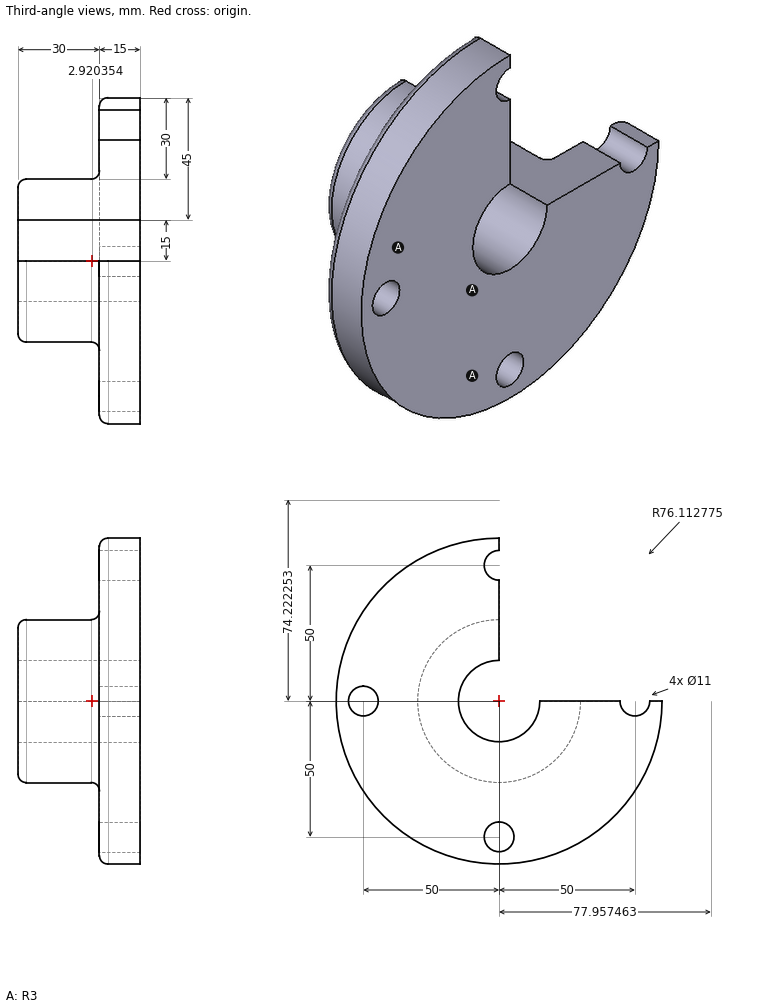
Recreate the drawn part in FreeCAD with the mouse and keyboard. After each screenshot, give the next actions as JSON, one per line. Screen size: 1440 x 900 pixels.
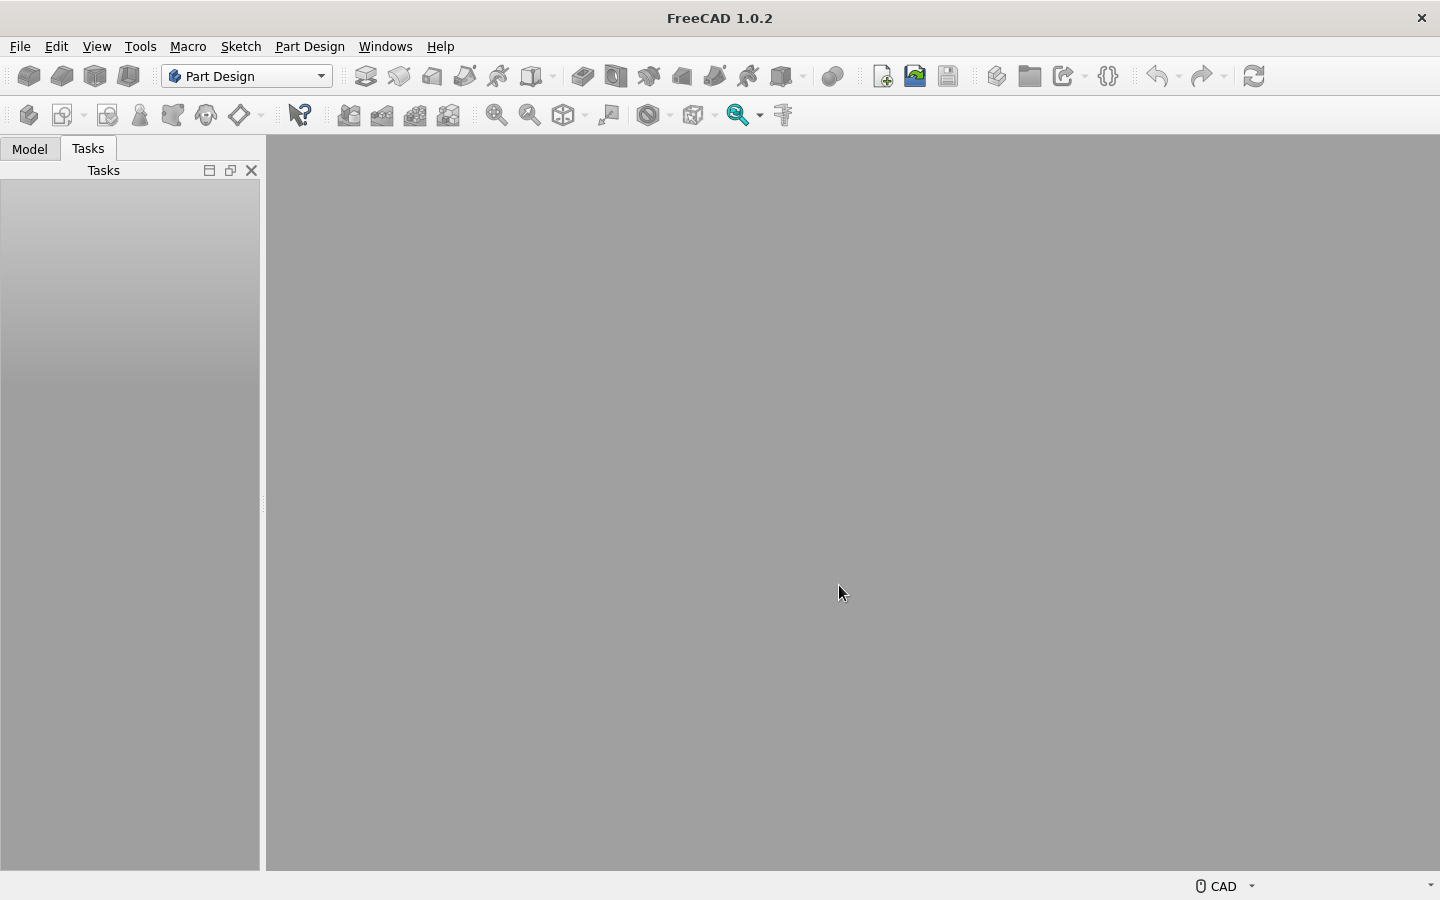
{"action": "left_click", "coordinate": [882, 76]}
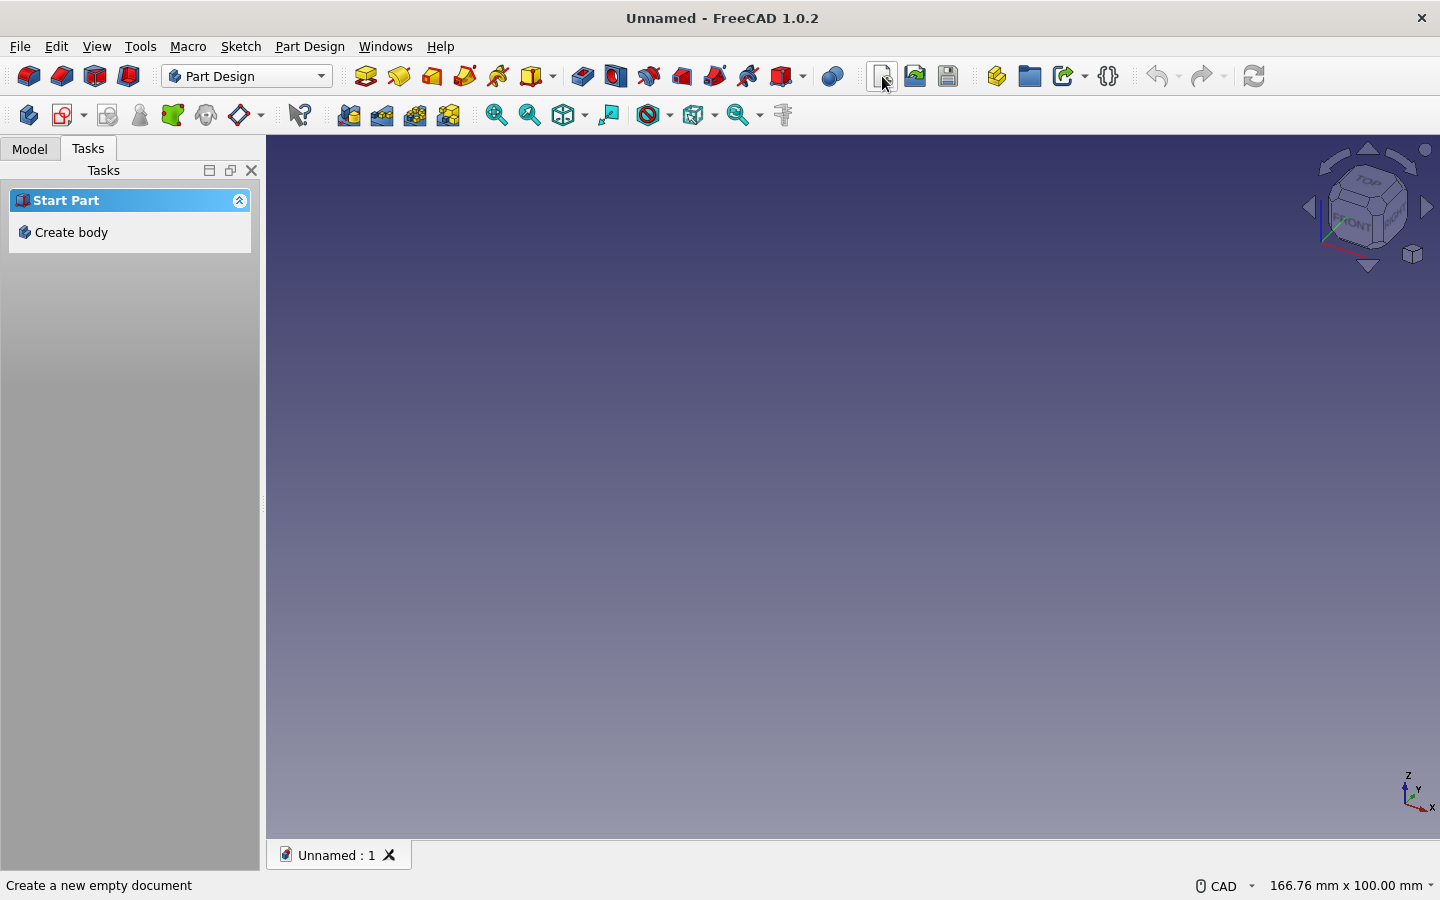
{"action": "left_click", "coordinate": [62, 116]}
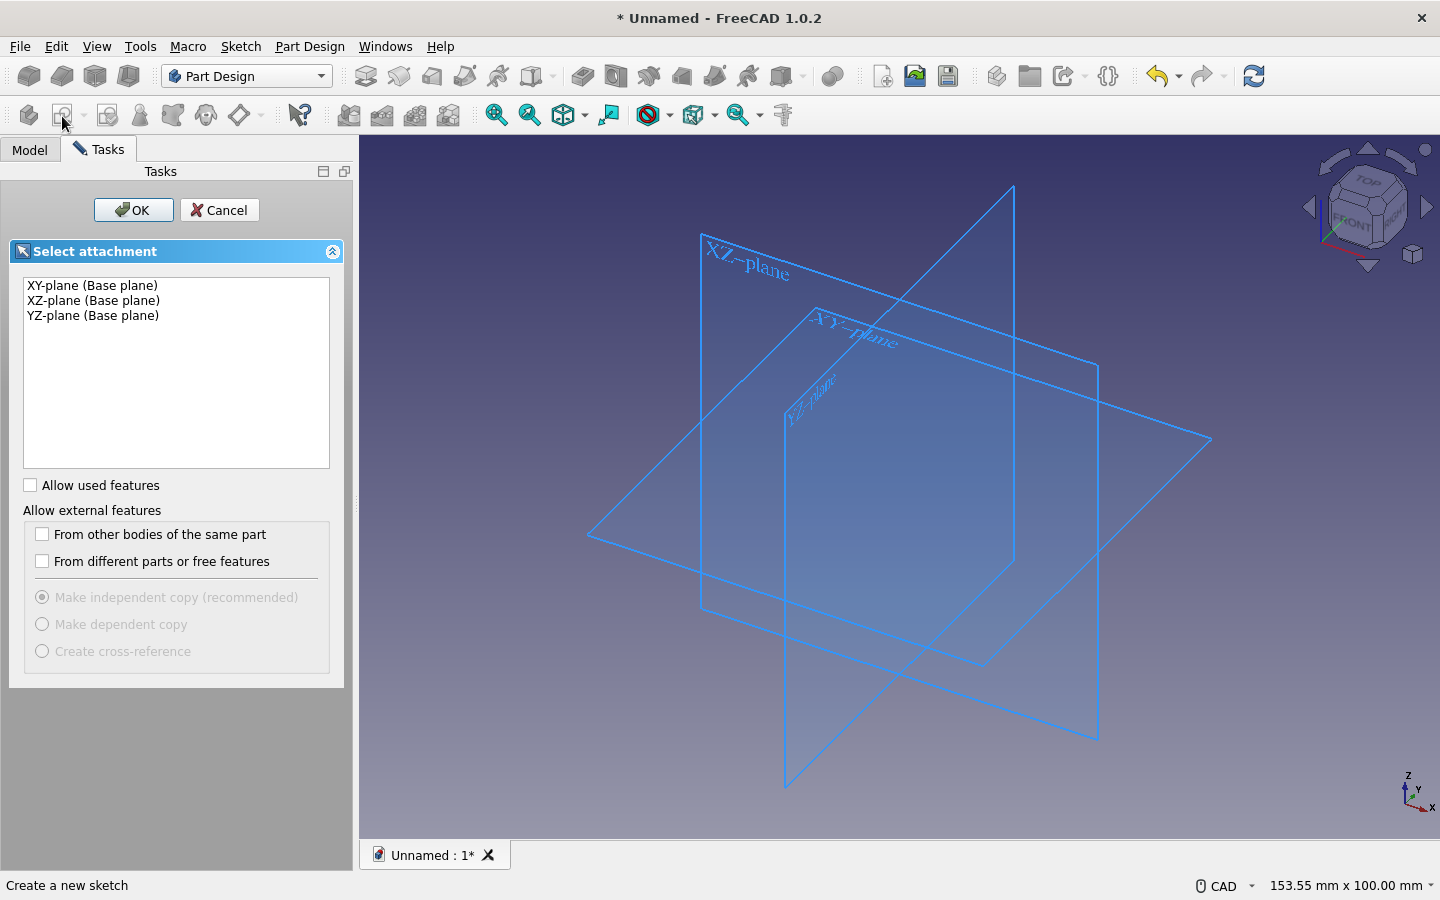
{"action": "left_click", "coordinate": [84, 286]}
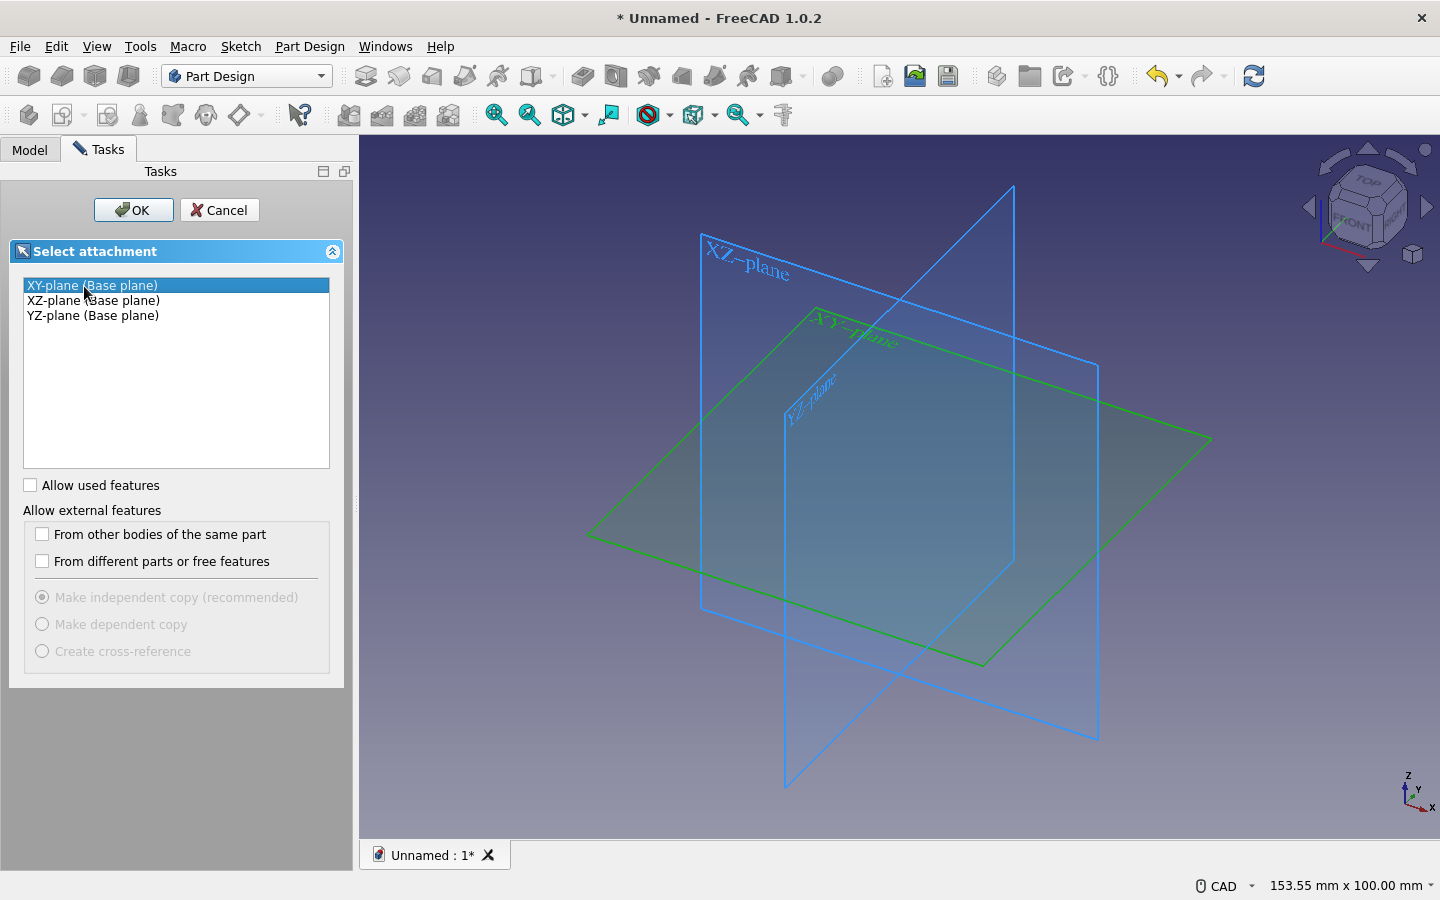
{"action": "left_click", "coordinate": [134, 210]}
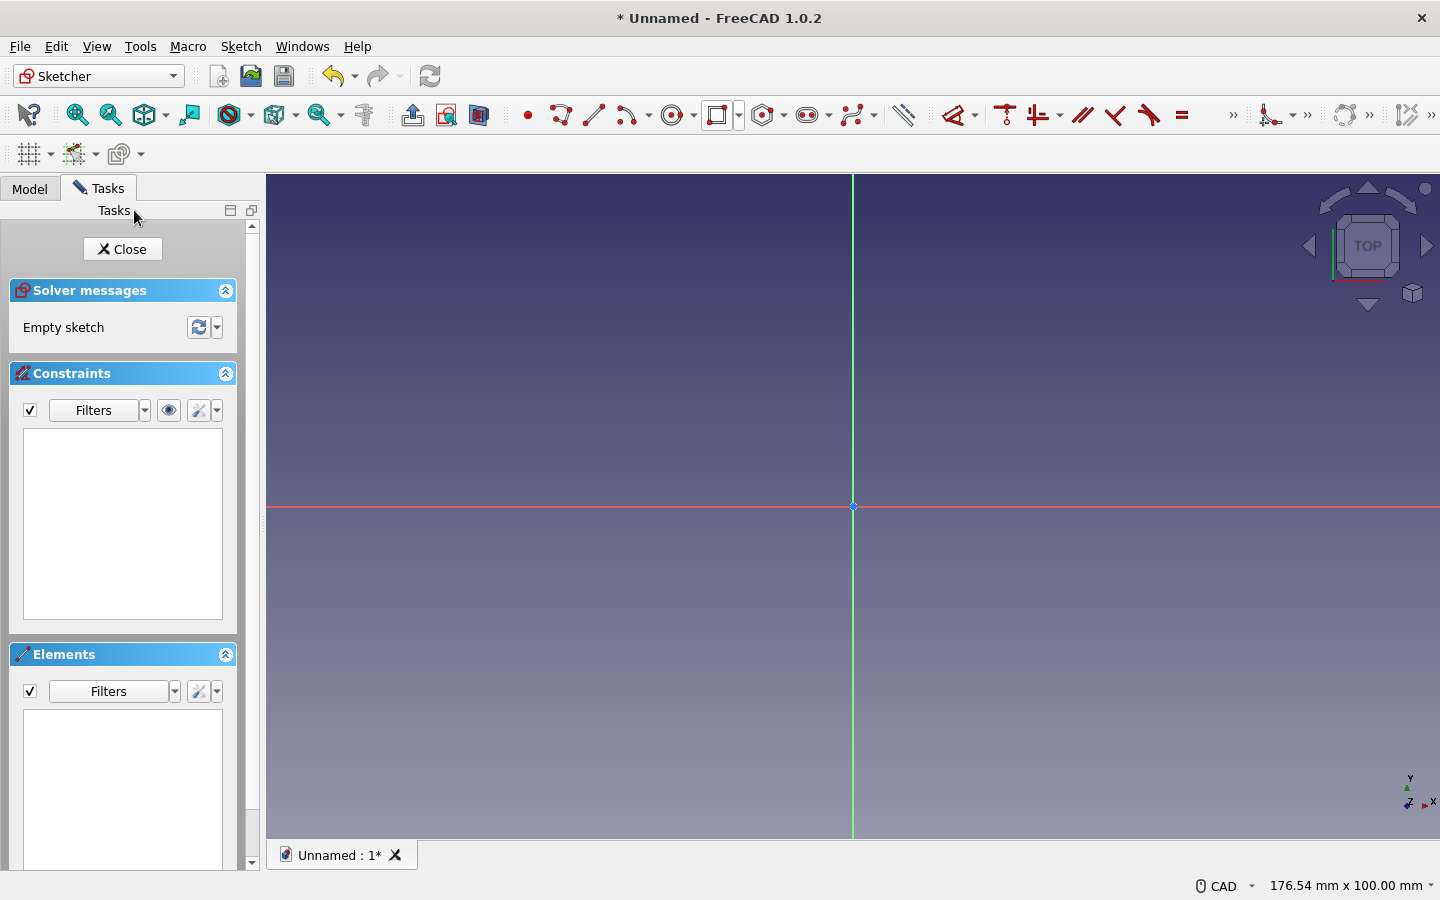
{"action": "scroll", "coordinate": [613, 811], "scroll_direction": "down", "scroll_amount": 1}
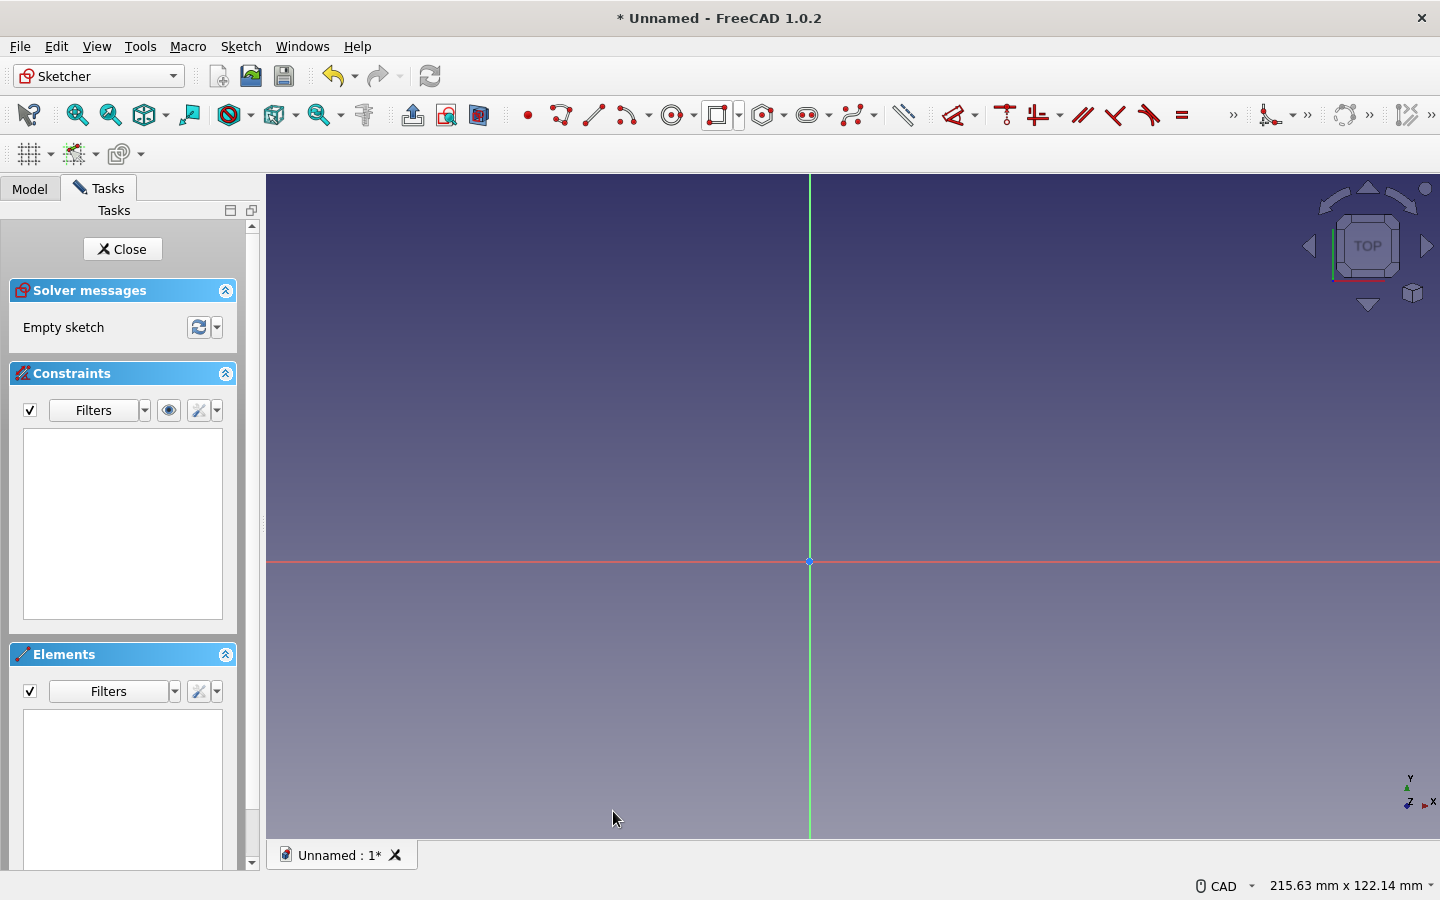
{"action": "left_click", "coordinate": [561, 116]}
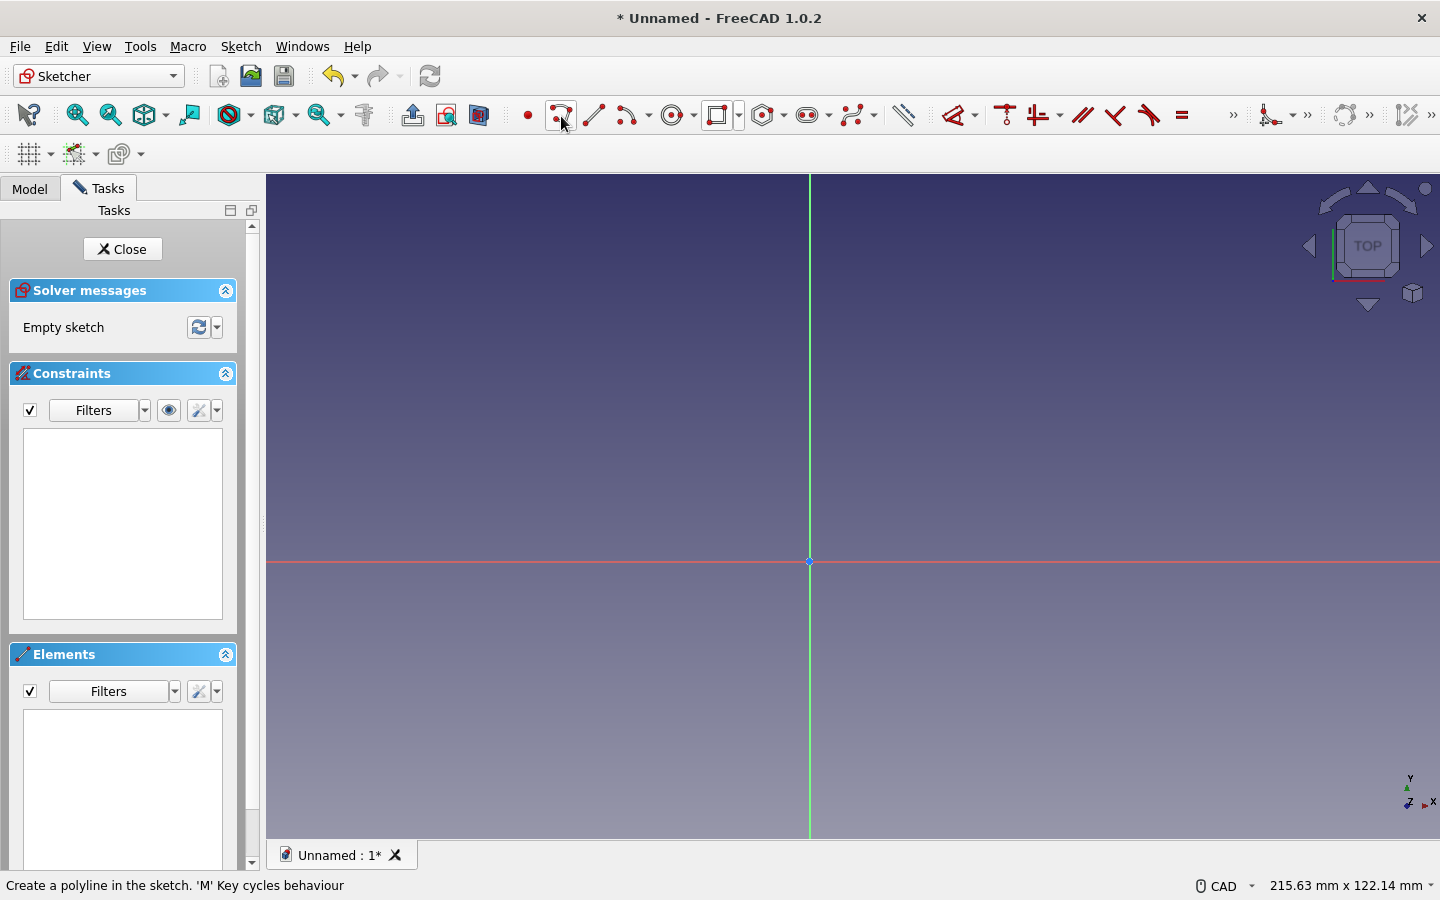
{"action": "left_click", "coordinate": [907, 480]}
{"action": "left_click", "coordinate": [907, 235]}
{"action": "left_click", "coordinate": [825, 235]}
{"action": "left_click", "coordinate": [825, 399]}
{"action": "left_click", "coordinate": [662, 399]}
{"action": "left_click", "coordinate": [662, 480]}
{"action": "left_click", "coordinate": [907, 481]}
{"action": "key", "text": "Escape"}
{"action": "key", "text": "Escape"}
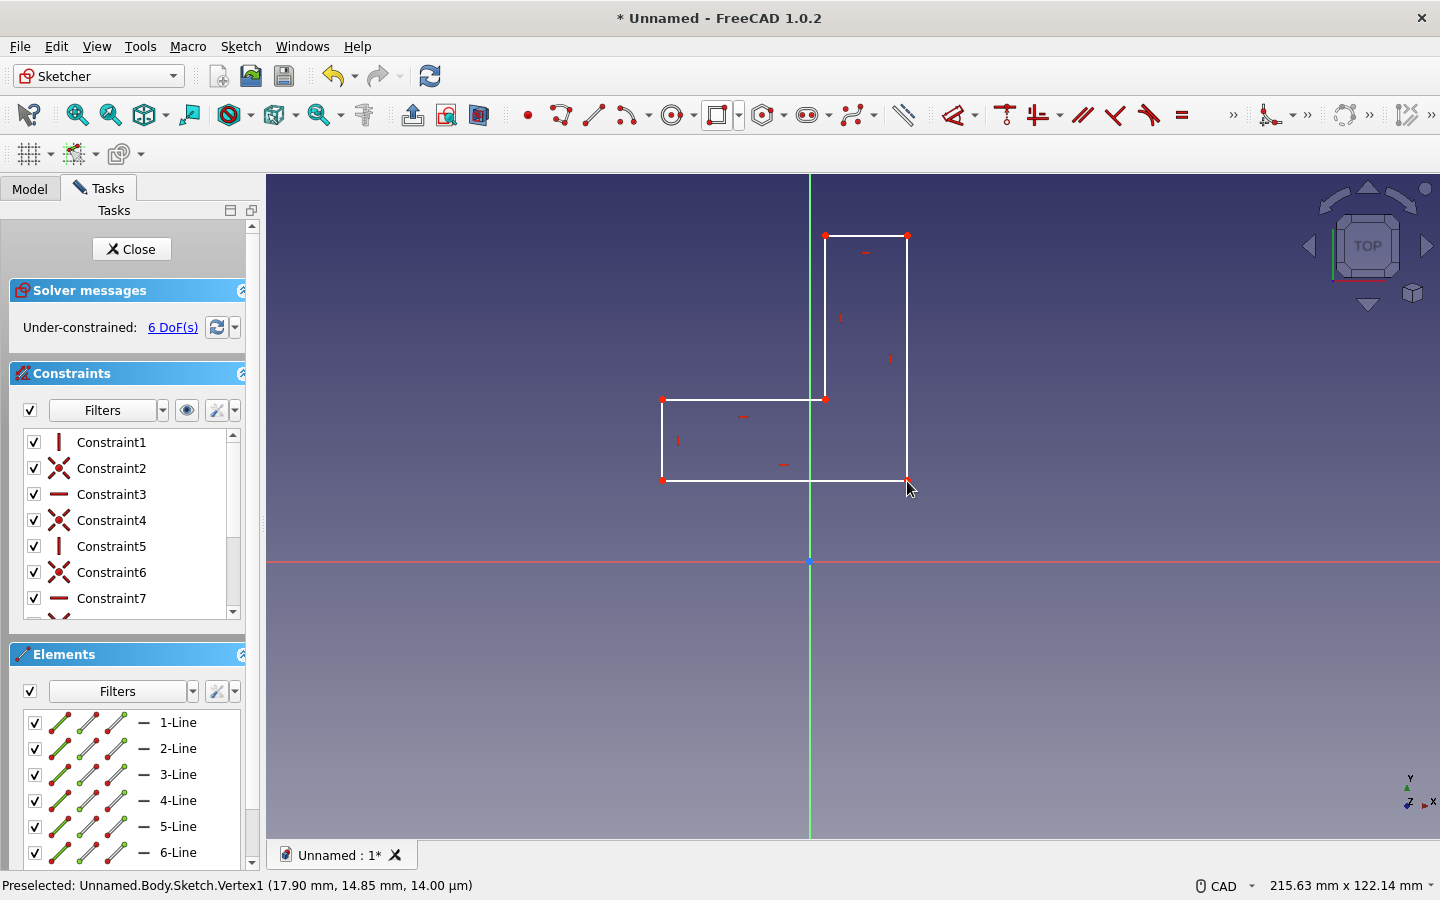
{"action": "left_click", "coordinate": [952, 116]}